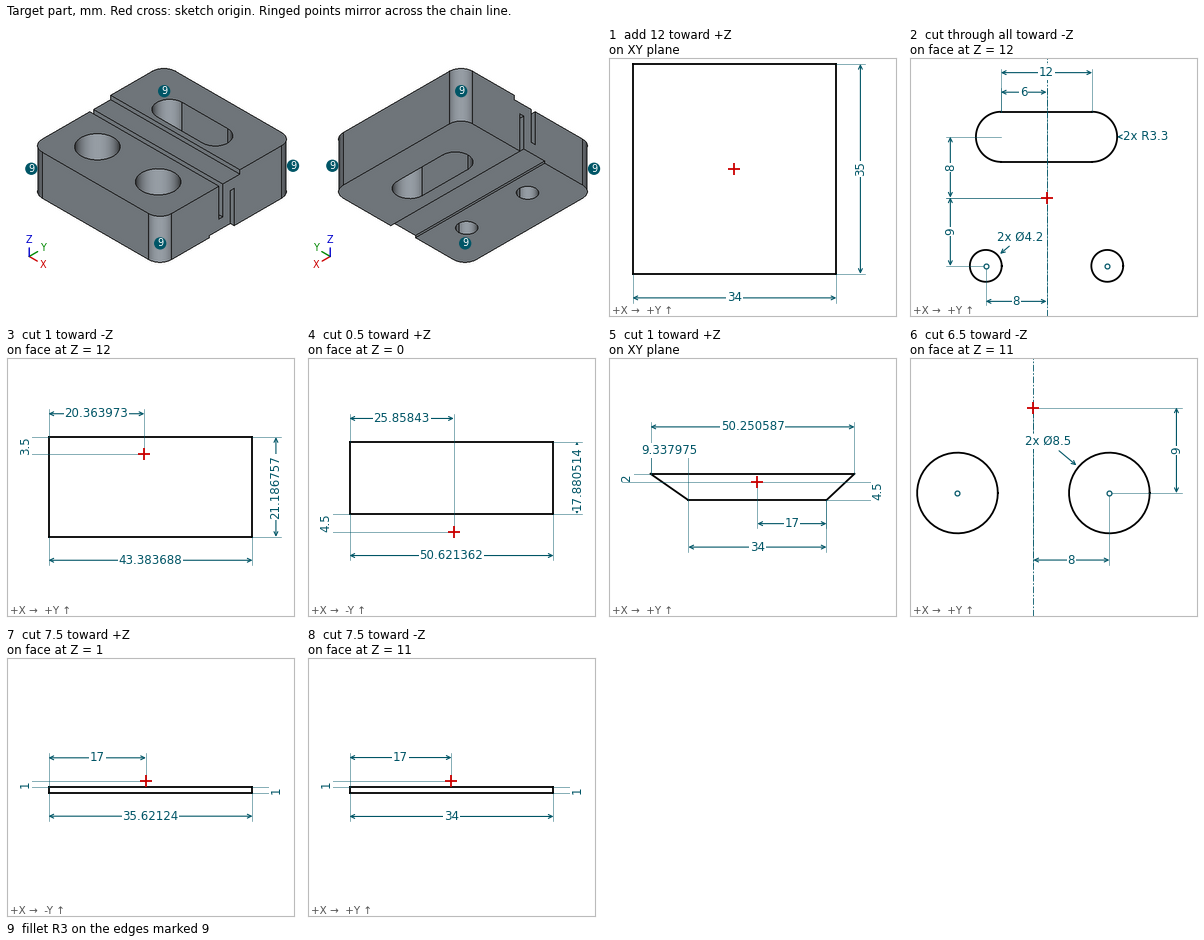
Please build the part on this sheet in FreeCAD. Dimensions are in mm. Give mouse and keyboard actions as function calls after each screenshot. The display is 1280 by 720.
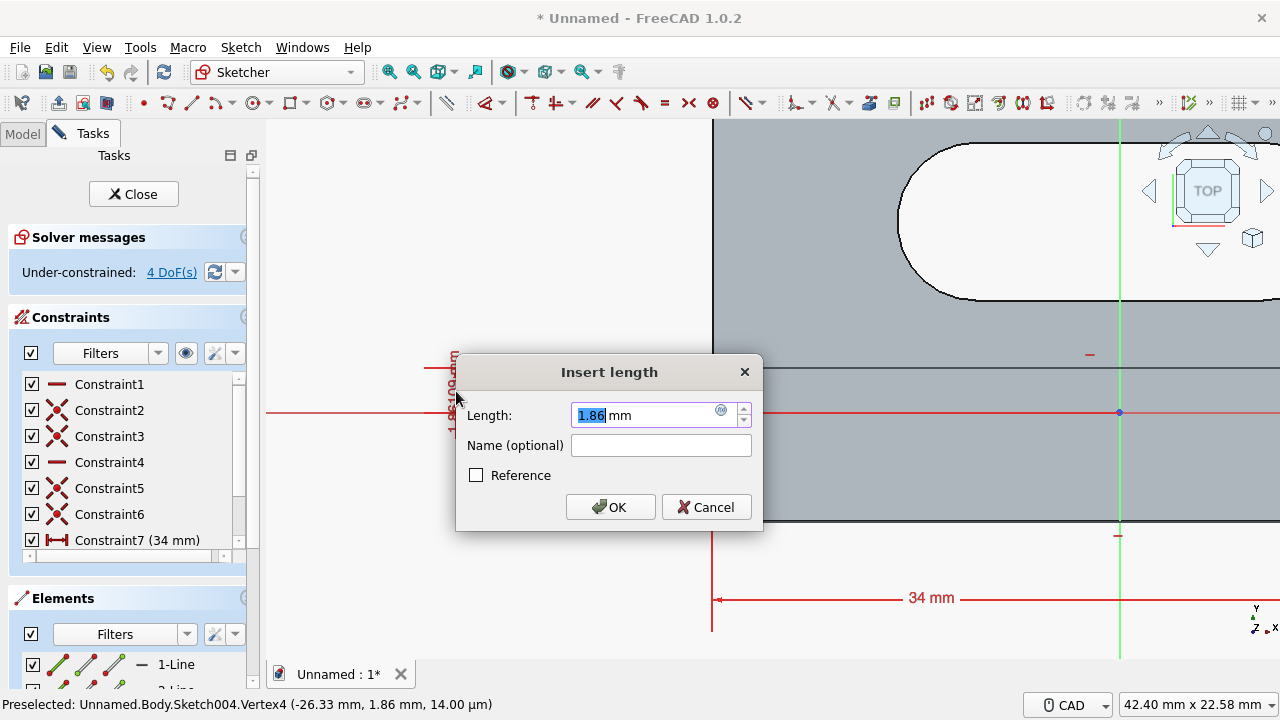
text(2)
key(Return)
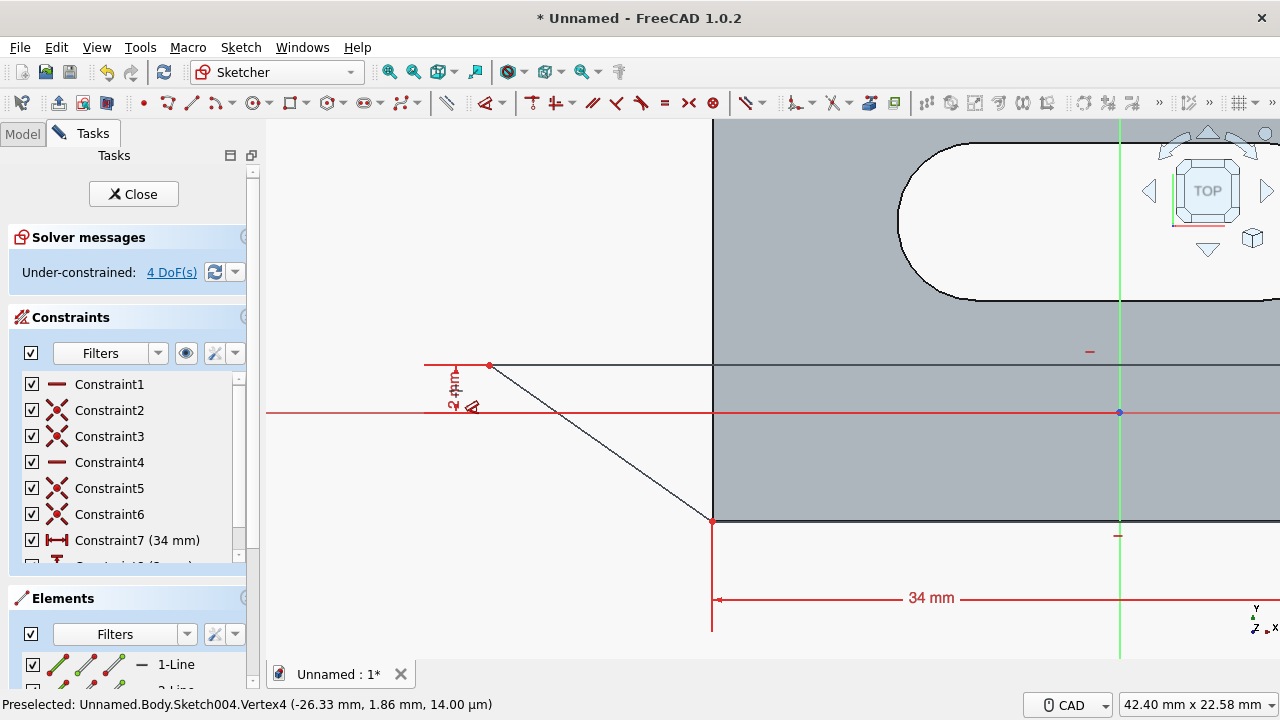
scroll(389, 345, down, 4)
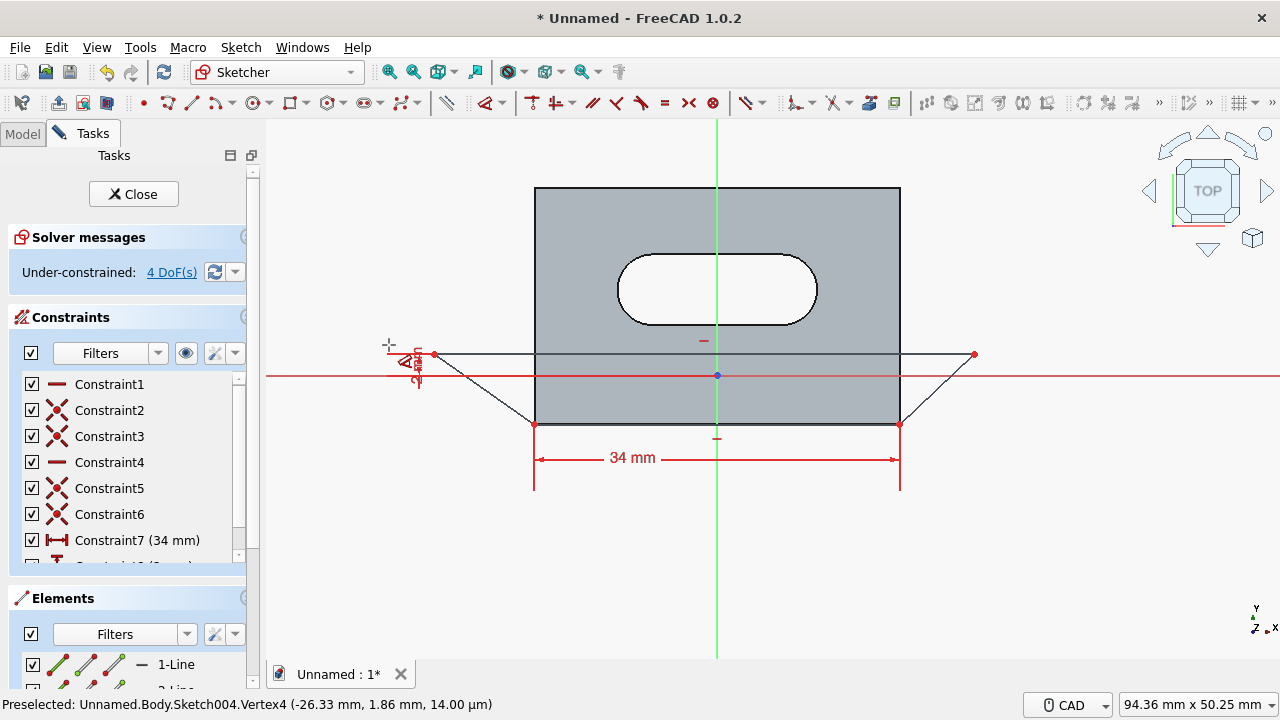
click(900, 425)
click(809, 459)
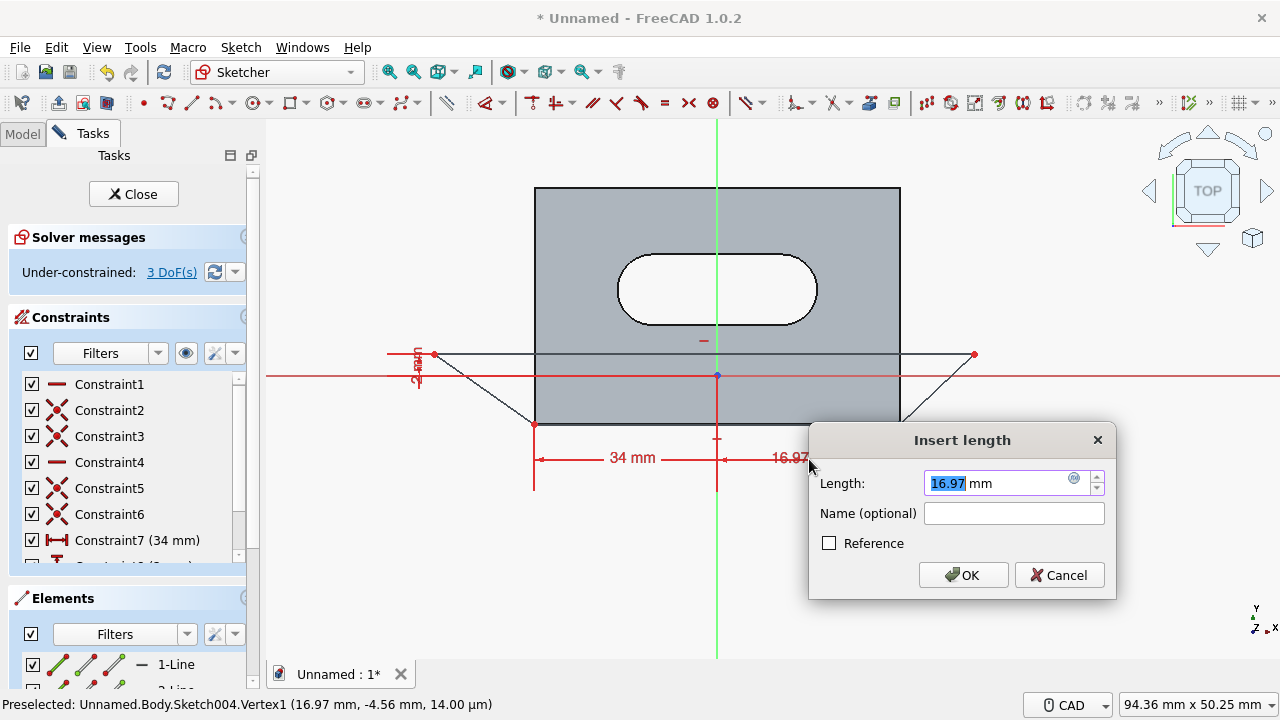
text(17)
key(Return)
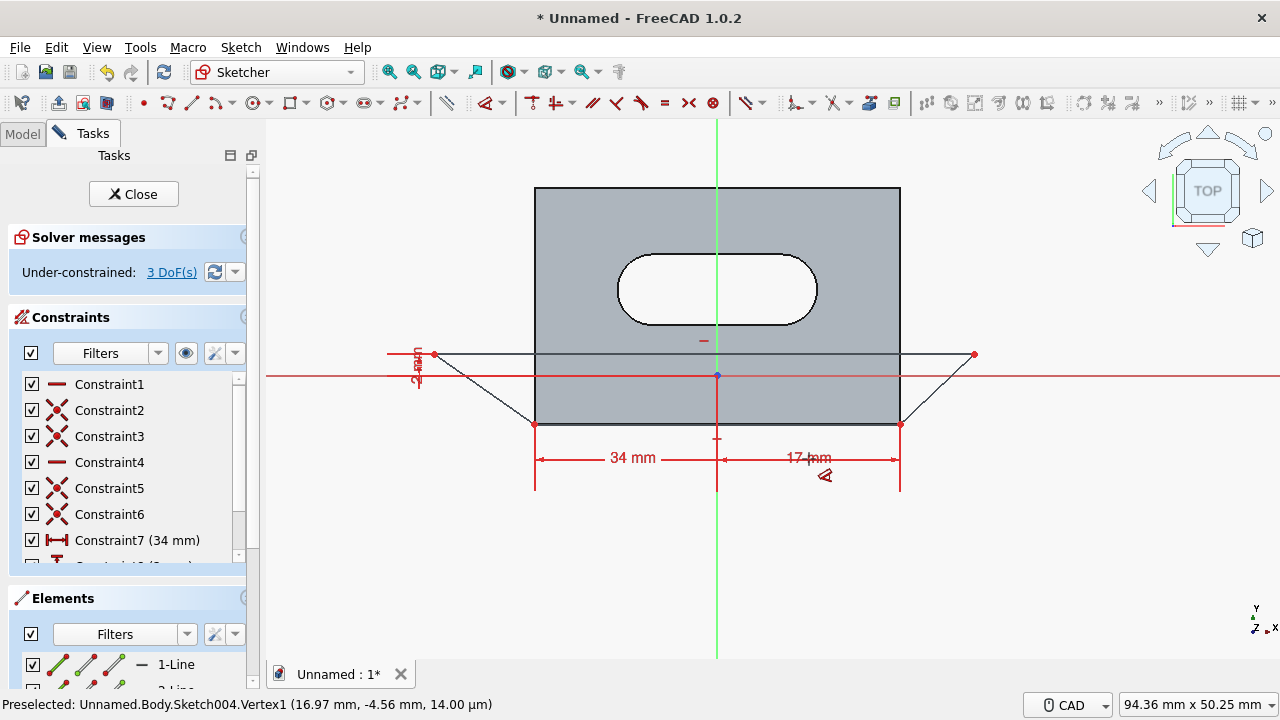
click(900, 425)
click(934, 412)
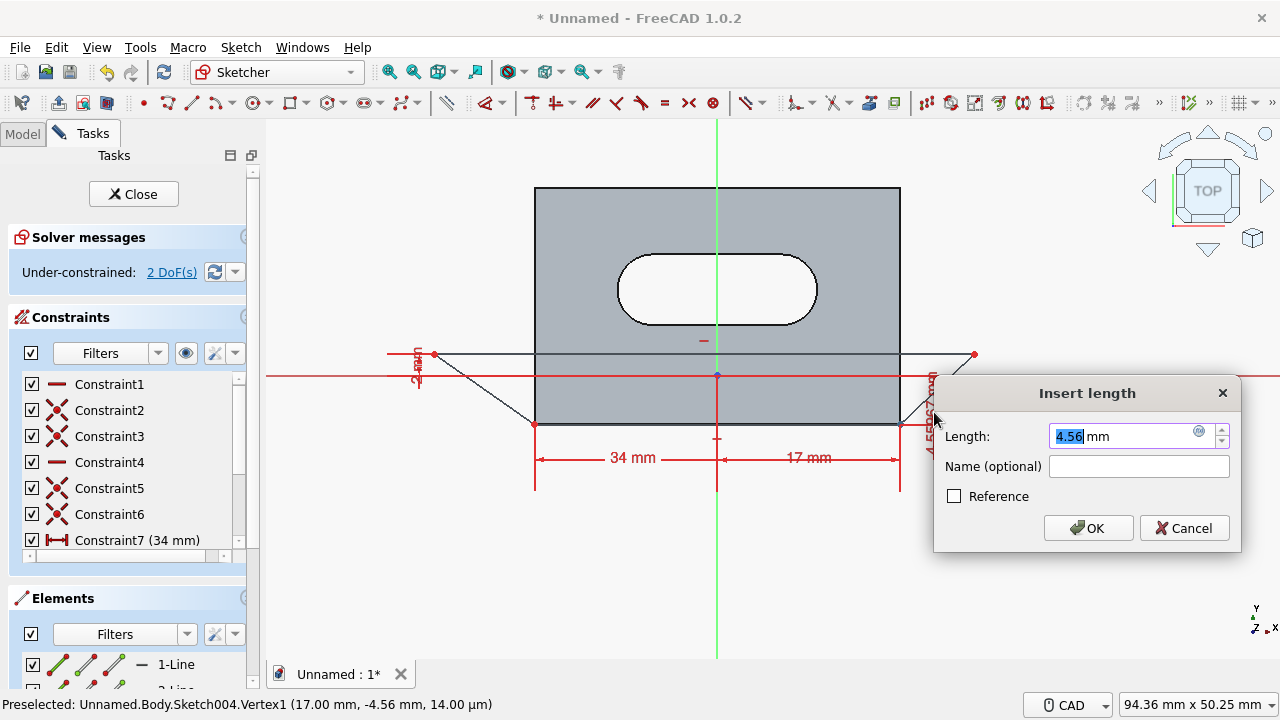
text(4.5)
key(Return)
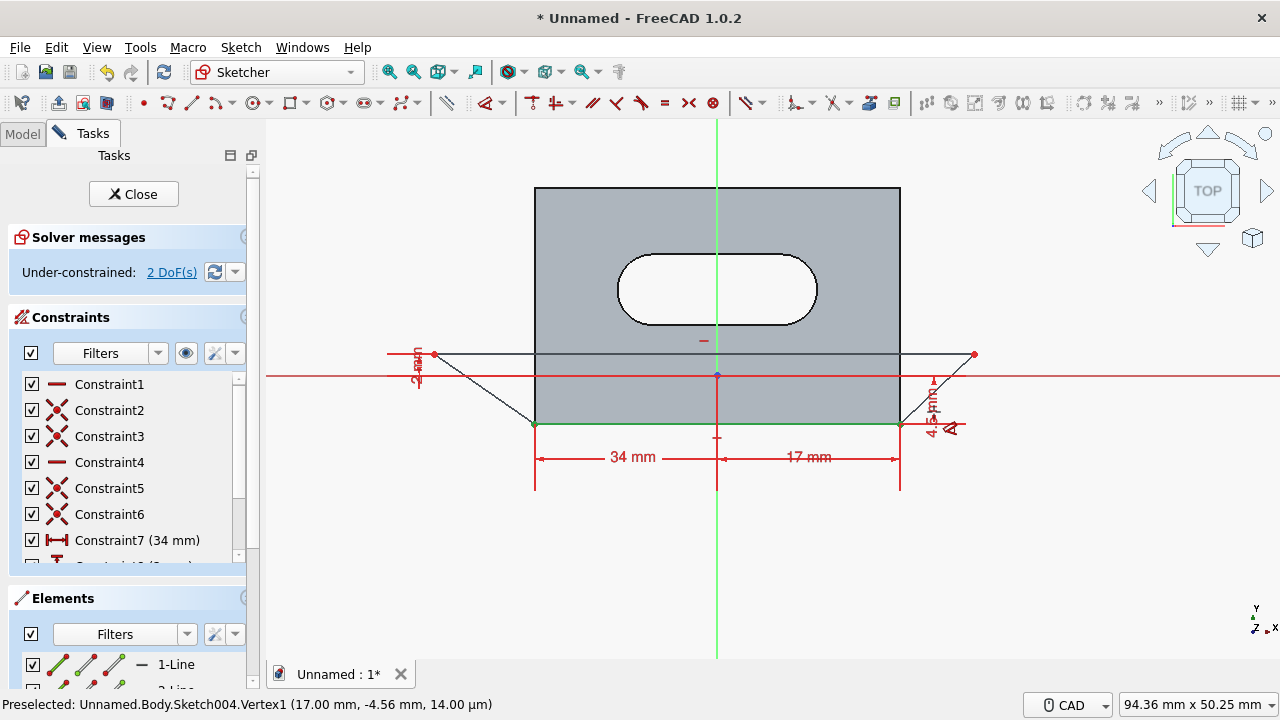
click(596, 354)
click(580, 320)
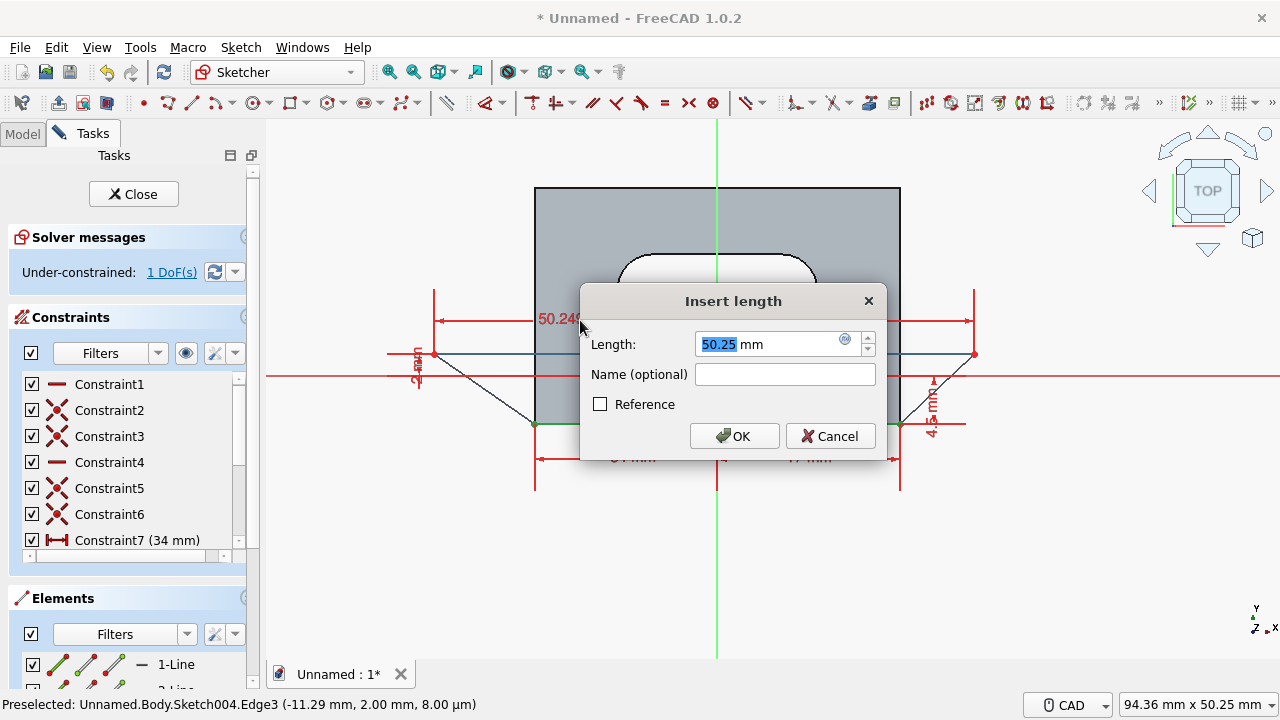
text(50.250587)
key(Return)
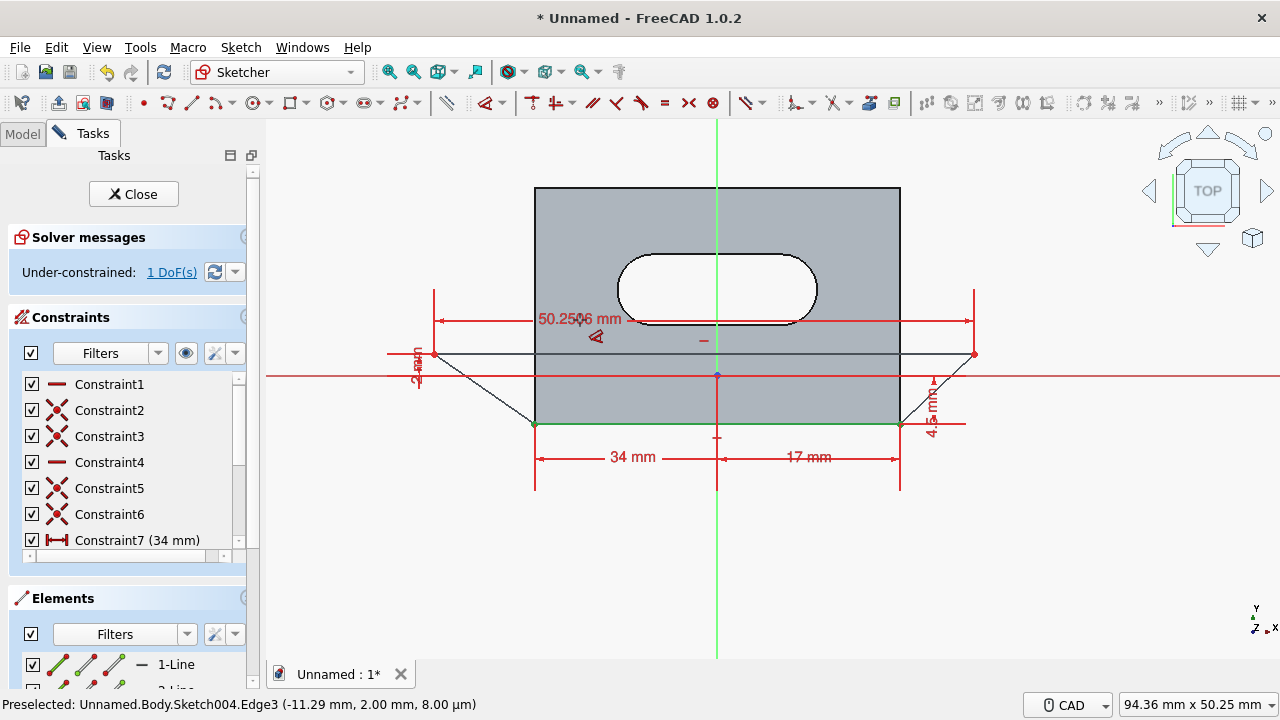
click(505, 403)
click(484, 458)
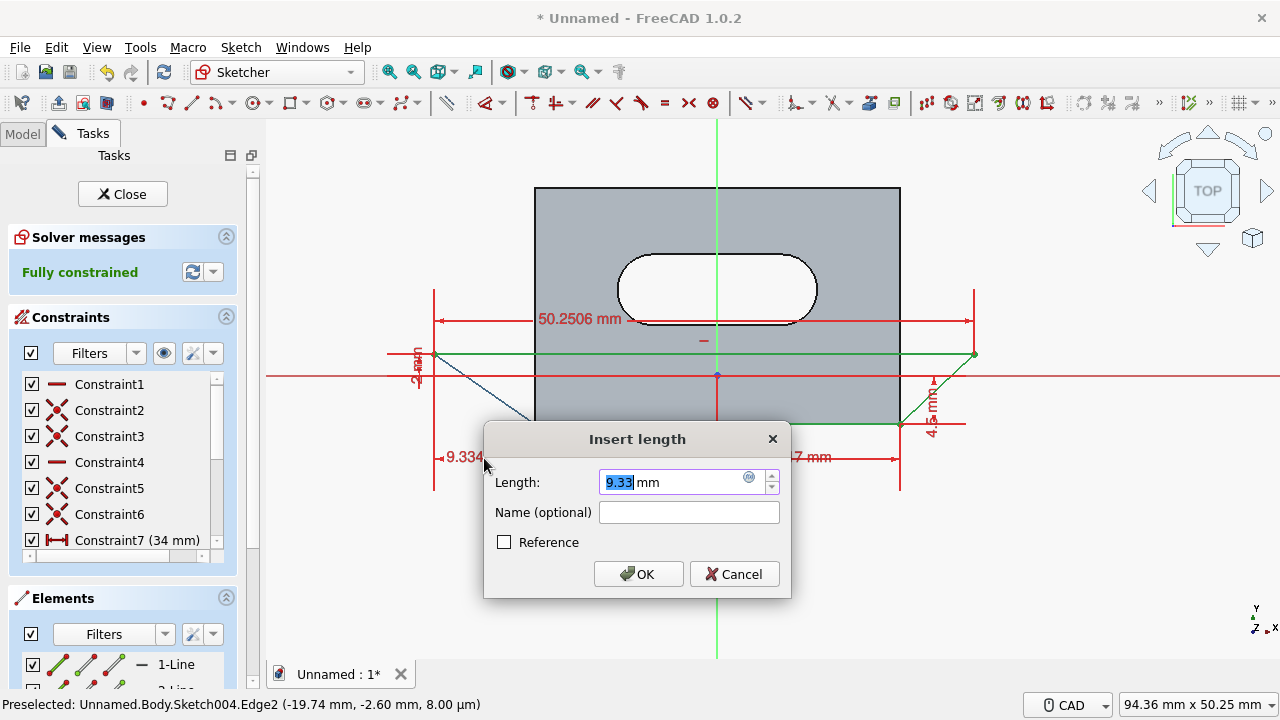
text(9.337975)
key(Return)
key(Escape)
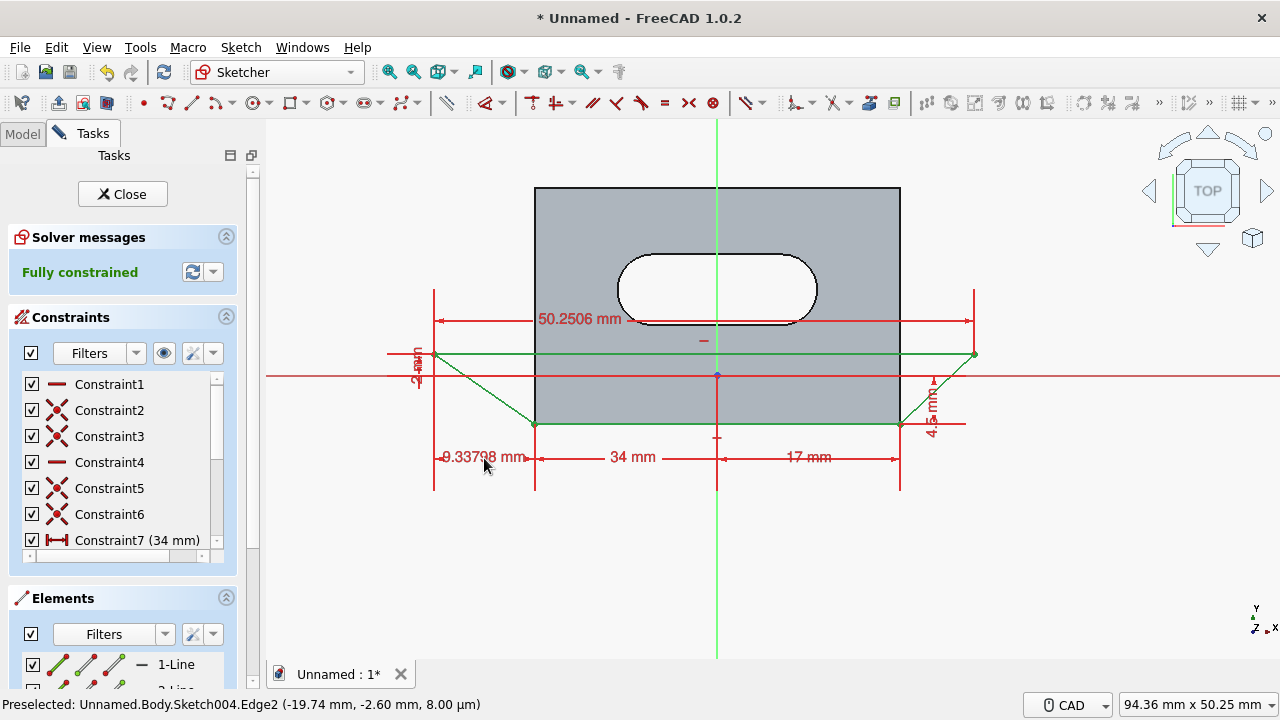
click(123, 194)